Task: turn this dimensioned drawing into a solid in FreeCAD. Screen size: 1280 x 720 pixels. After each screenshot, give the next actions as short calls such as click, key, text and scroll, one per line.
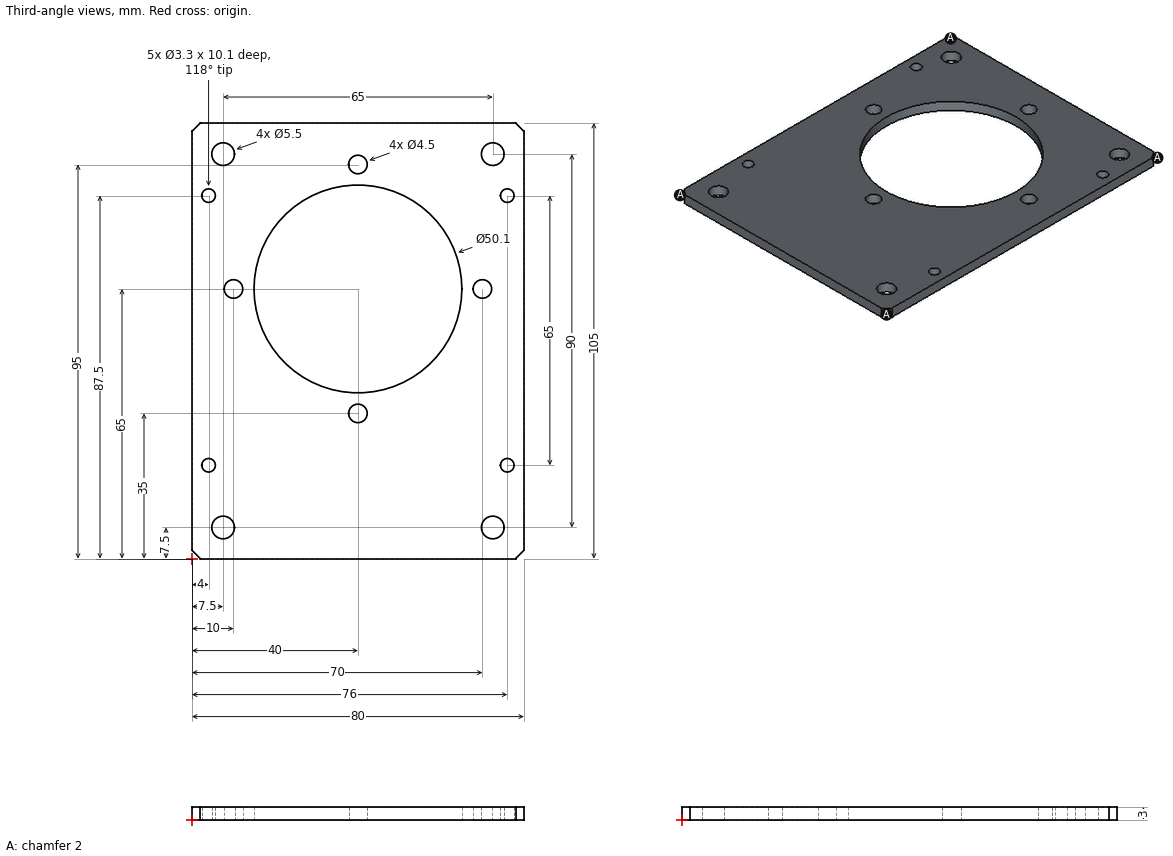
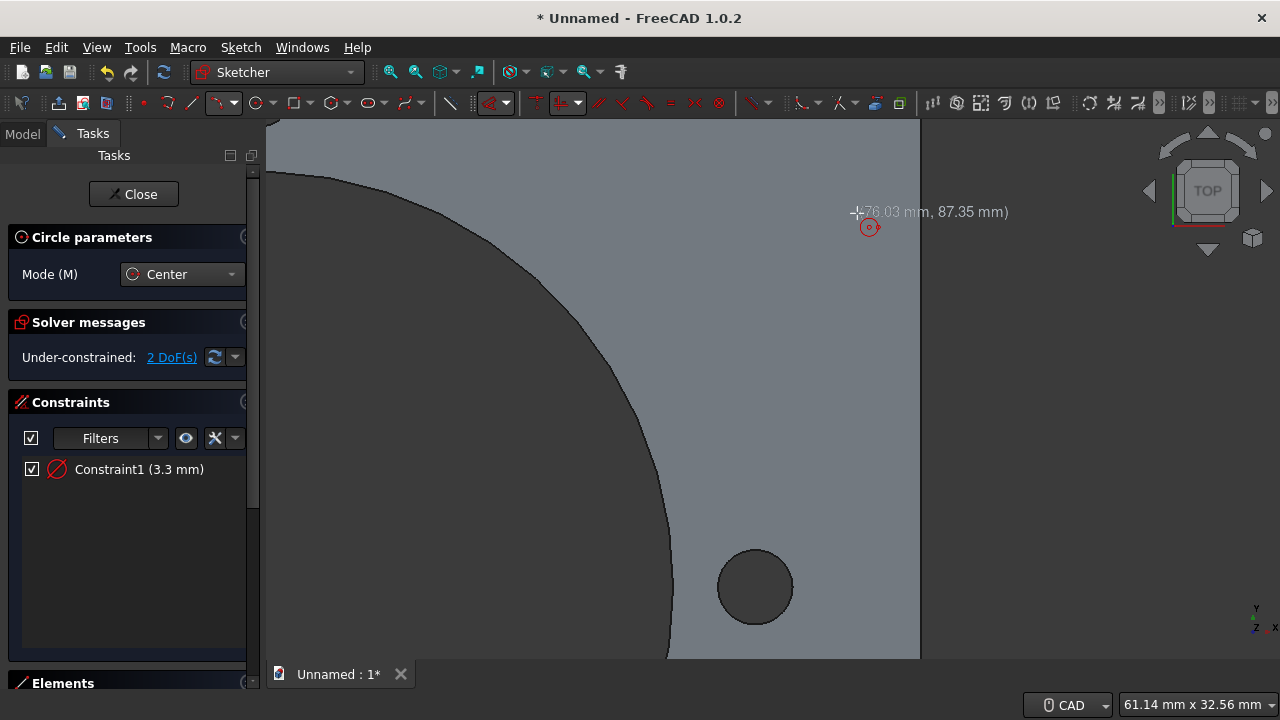
scroll(857, 213, down, 7)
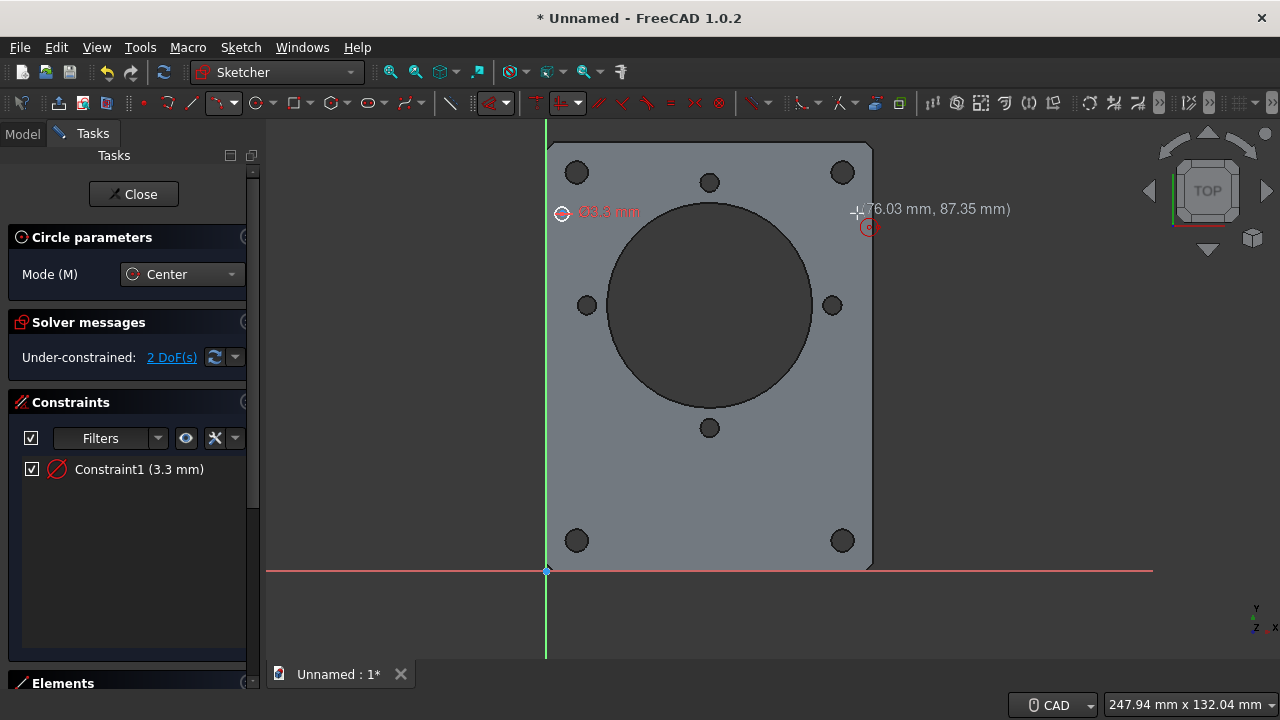
click(857, 213)
move(862, 209)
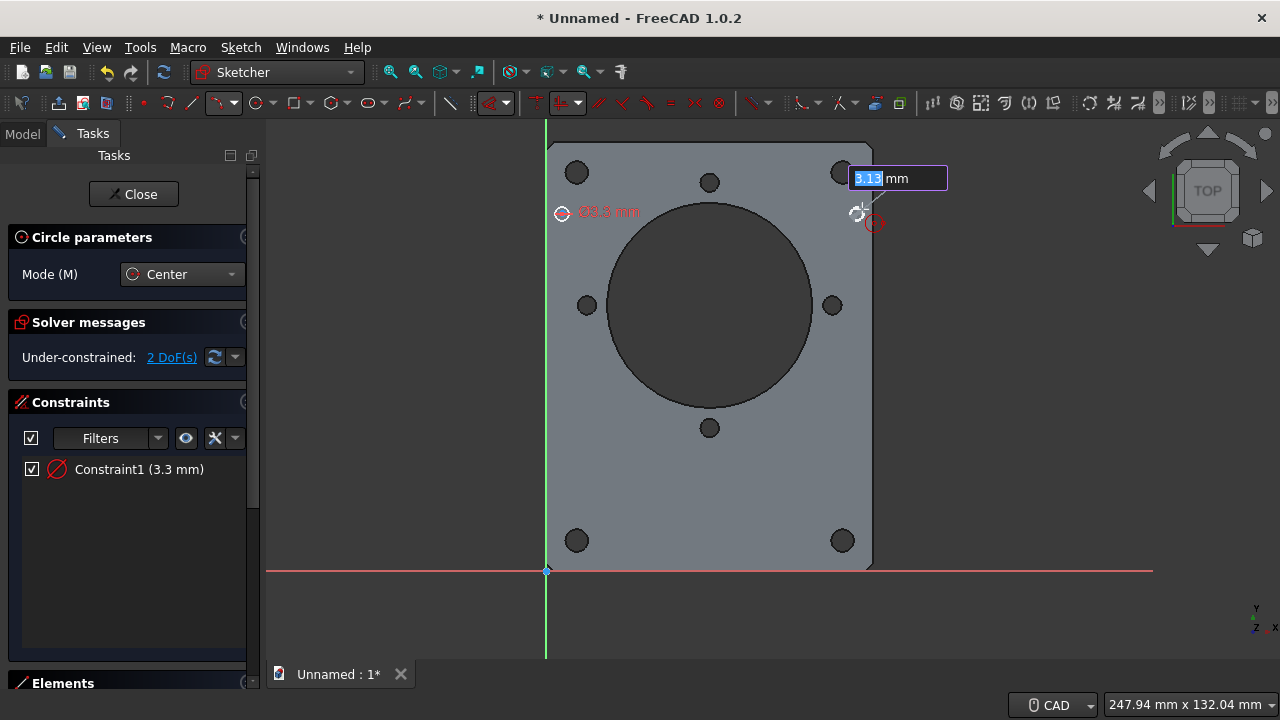
text(3.3)
key(Return)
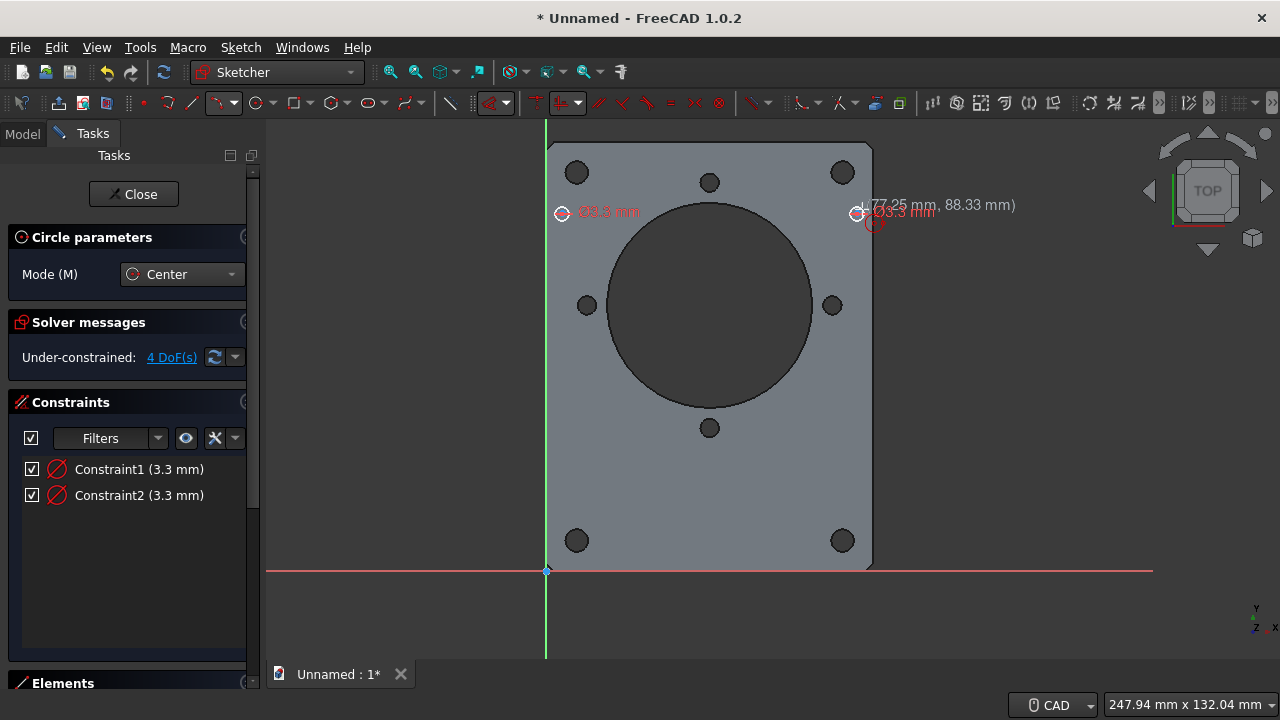
scroll(857, 479, up, 7)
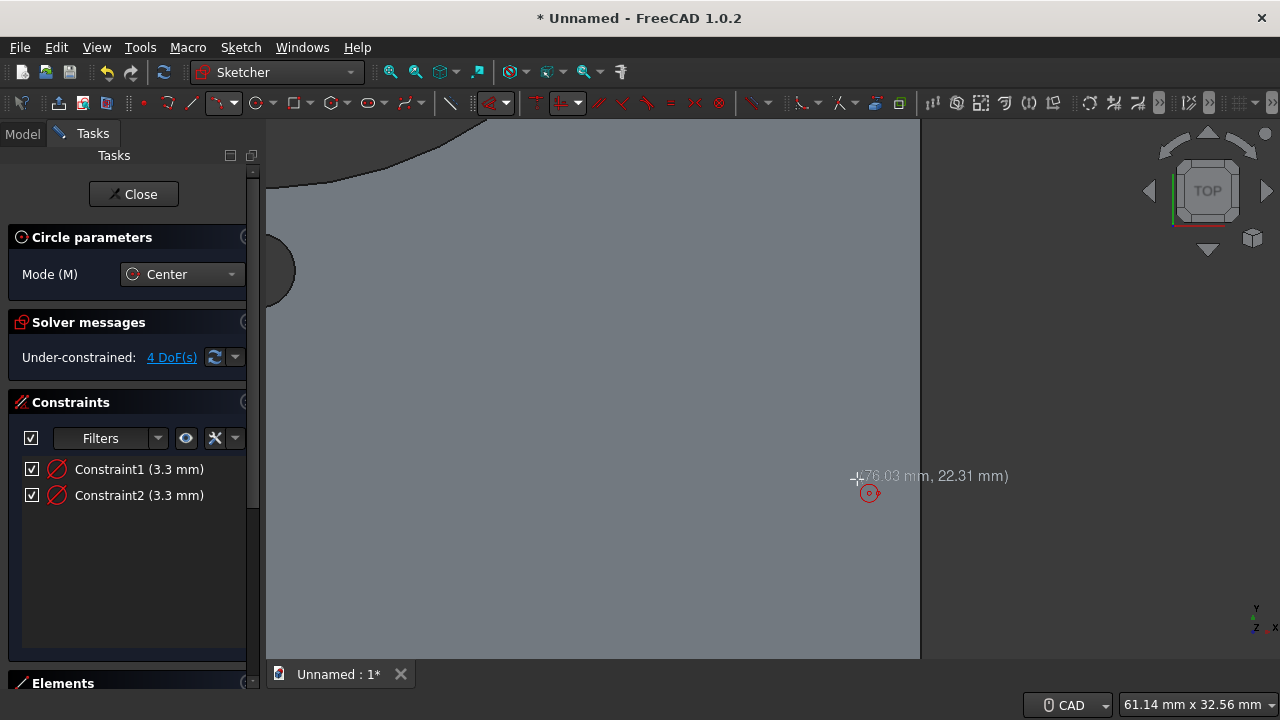
scroll(857, 480, down, 7)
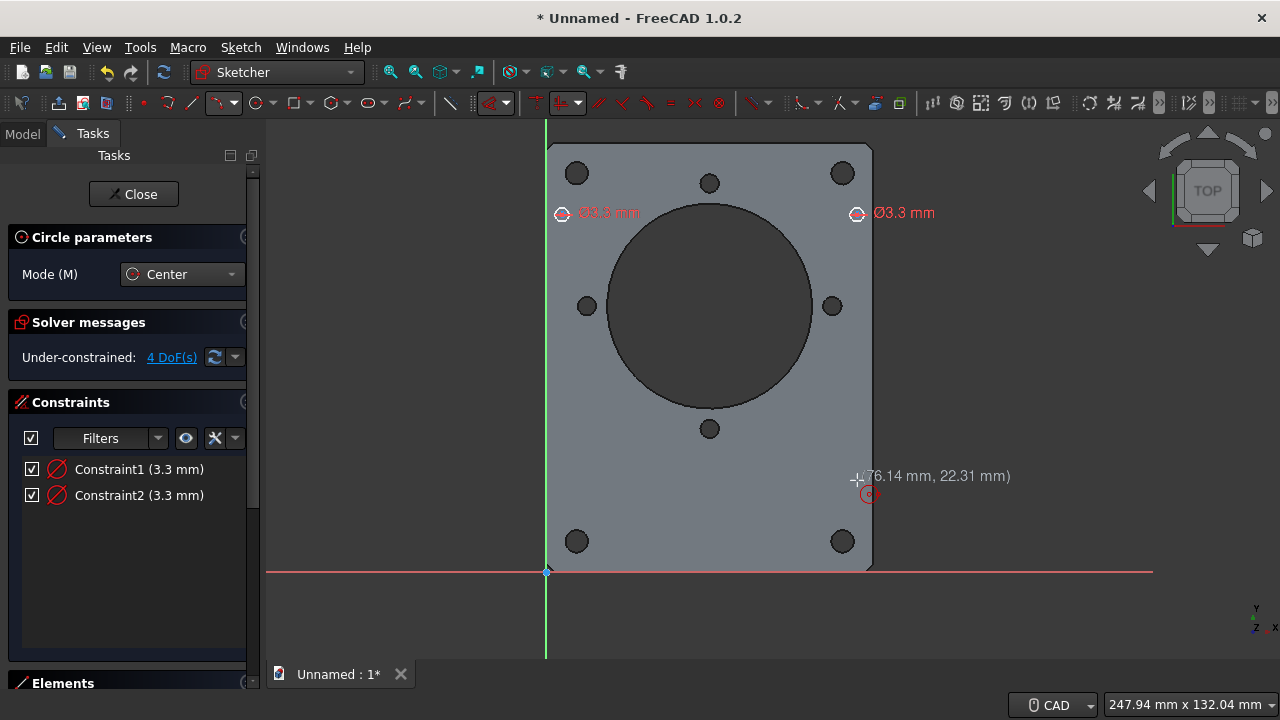
click(857, 480)
move(862, 475)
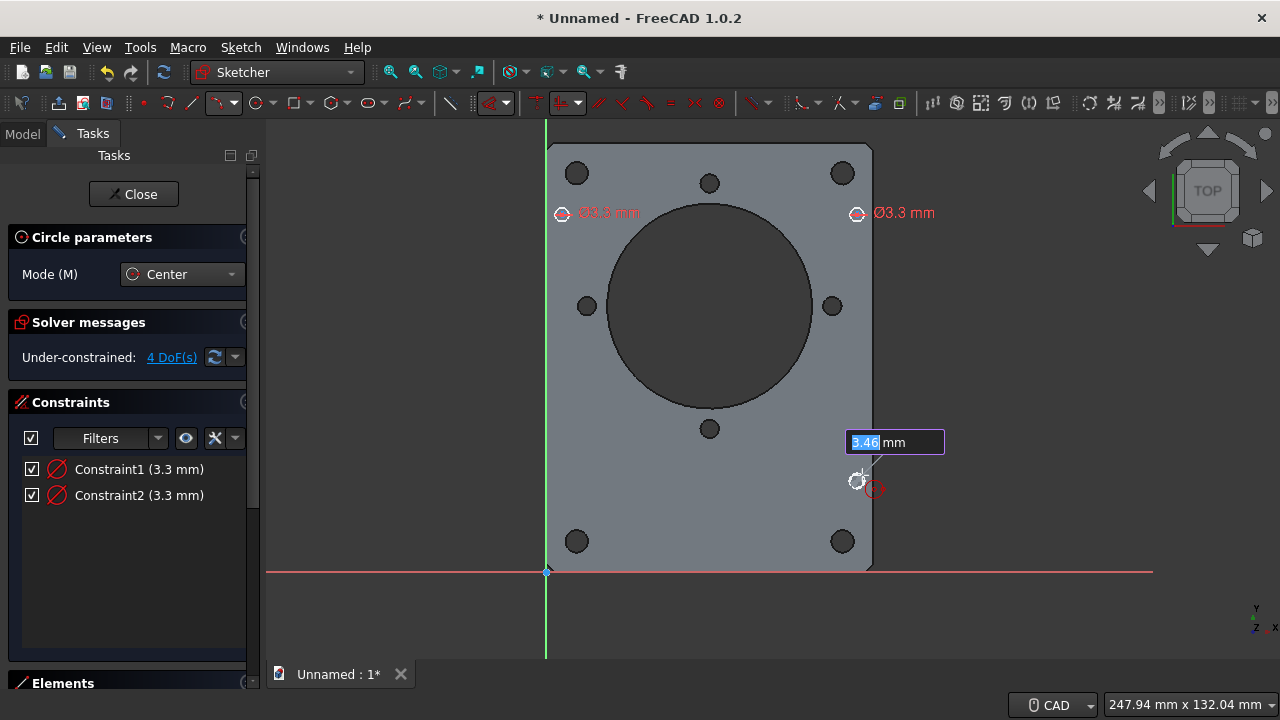
text(3.3)
key(Return)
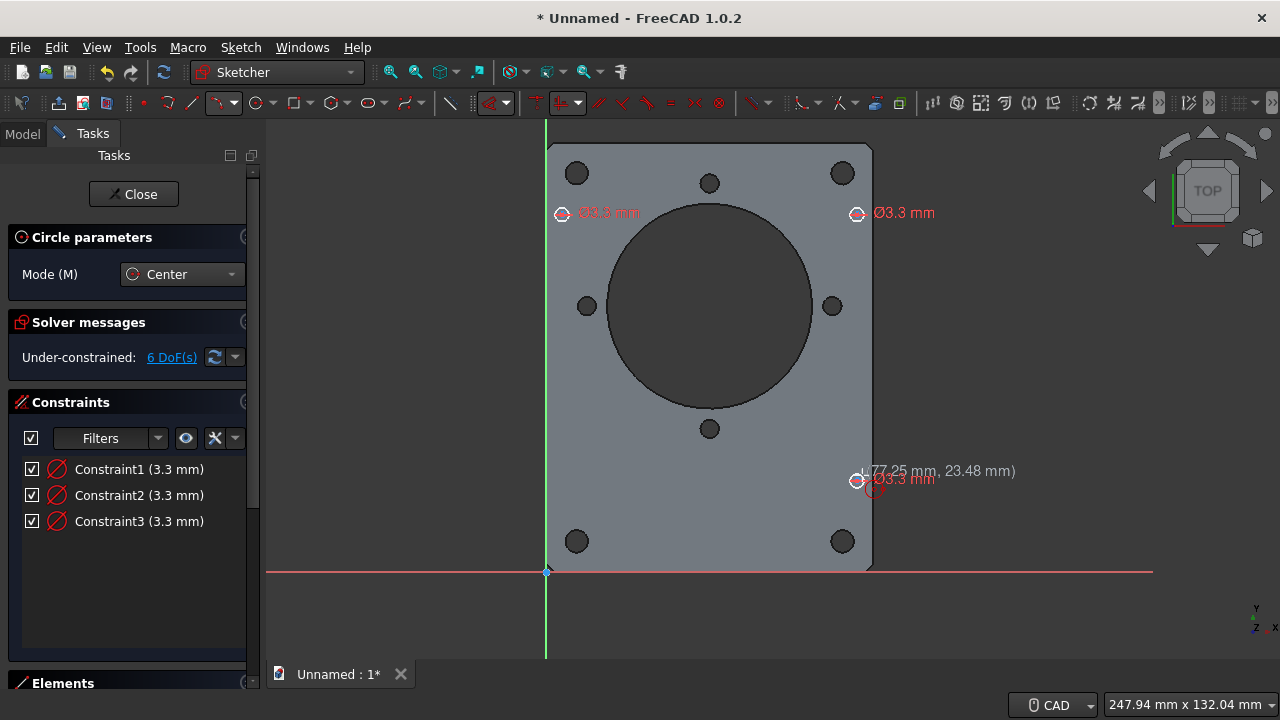
scroll(562, 480, up, 7)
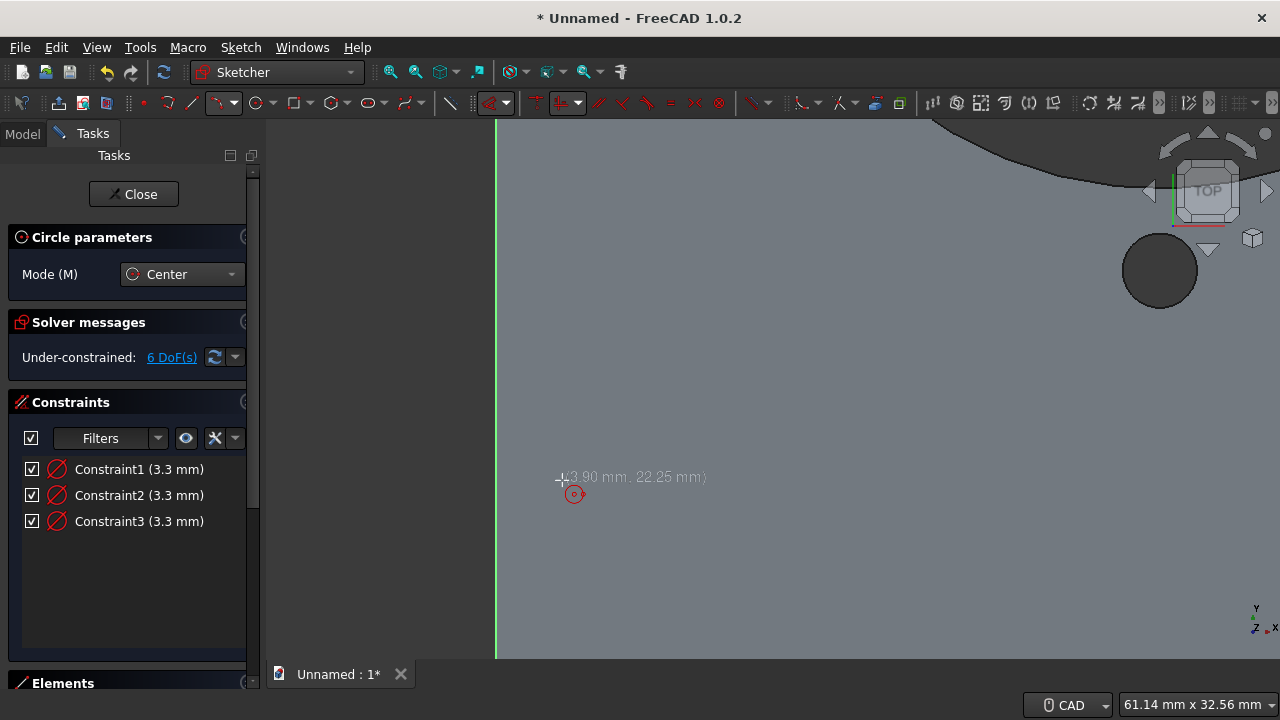
scroll(562, 480, down, 7)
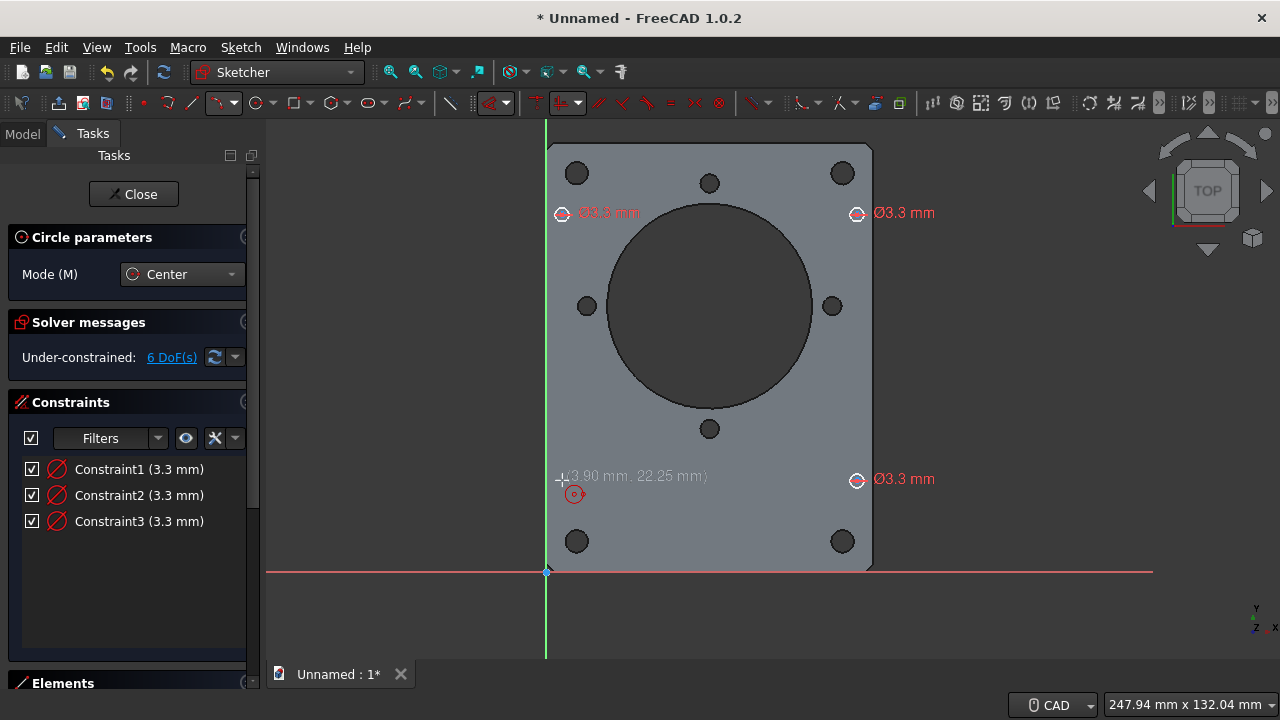
click(562, 480)
move(567, 475)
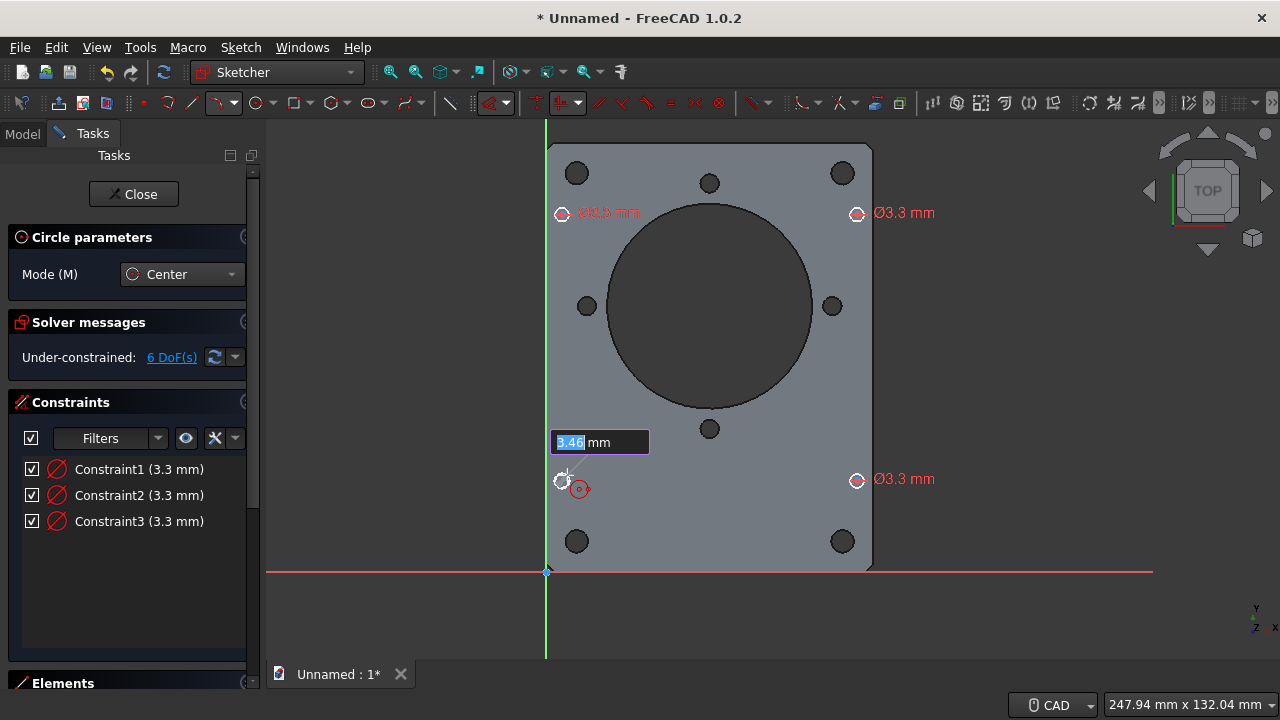
text(3.3)
key(Return)